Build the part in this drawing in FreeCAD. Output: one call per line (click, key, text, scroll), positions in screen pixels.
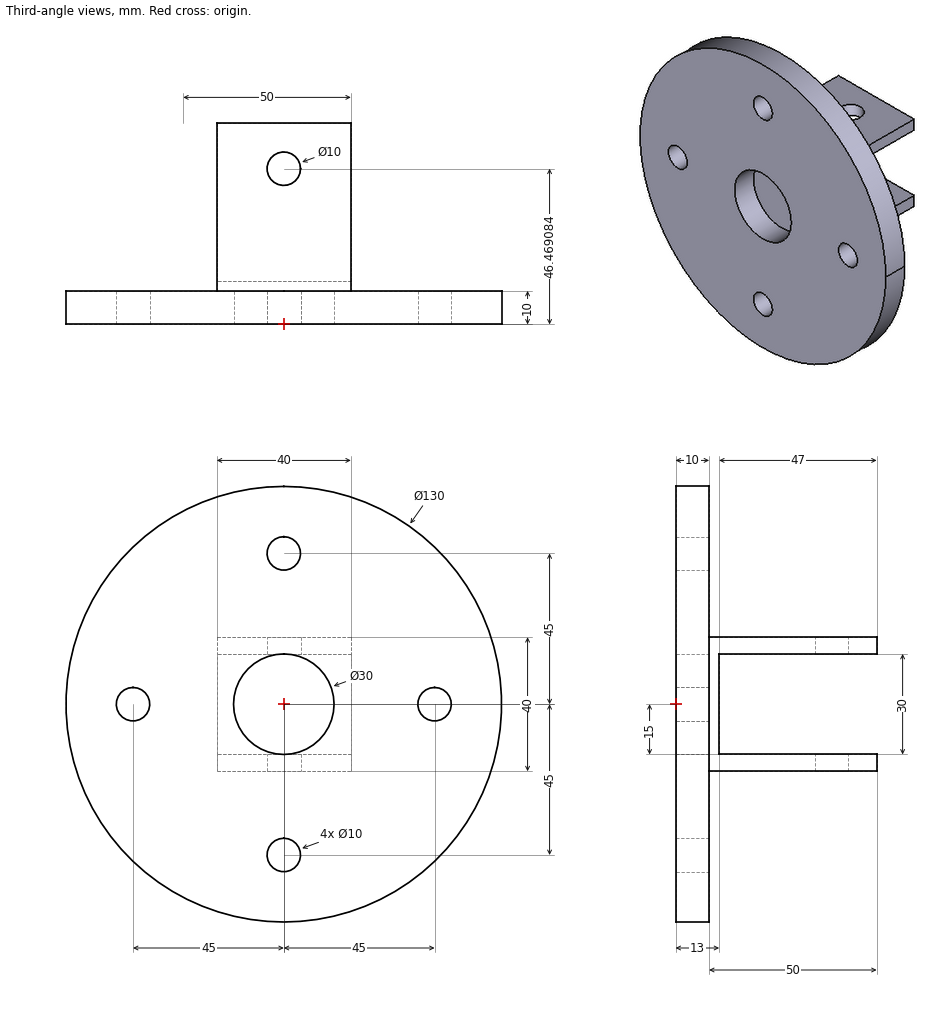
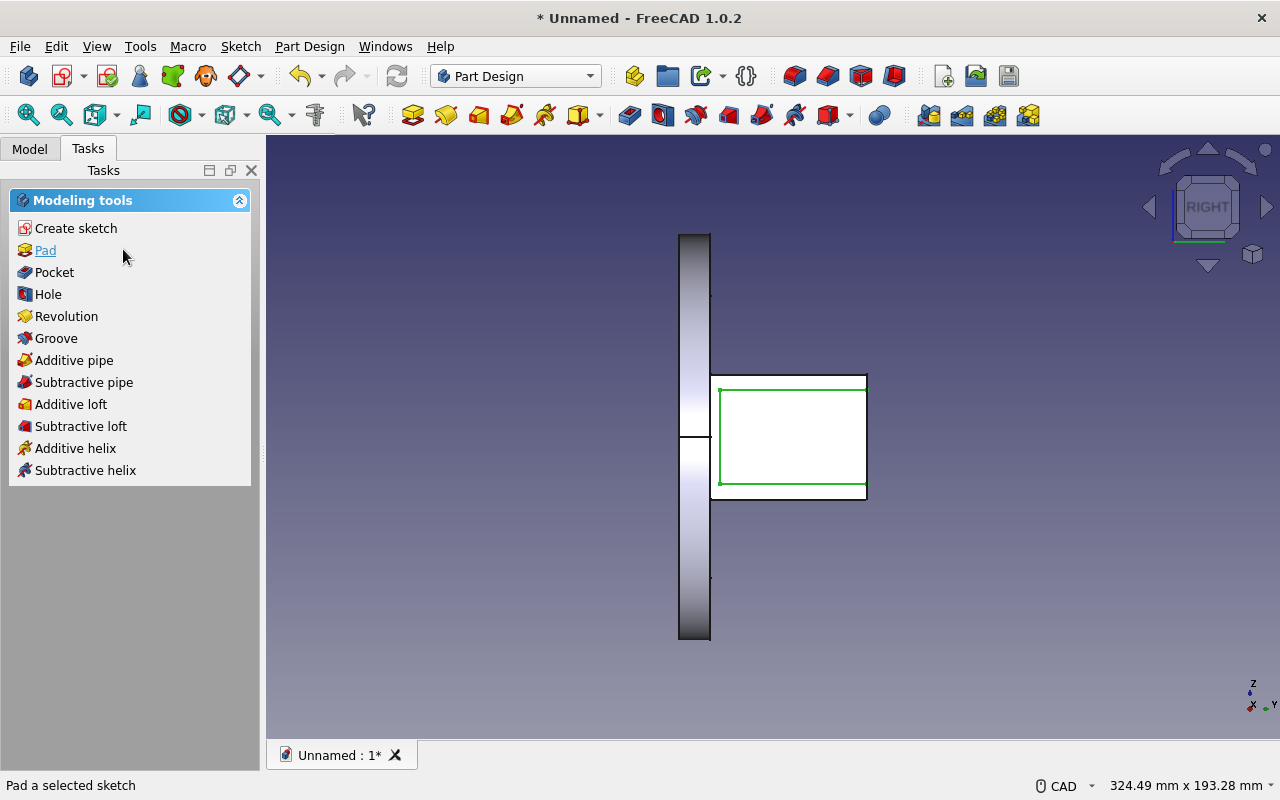
click(630, 116)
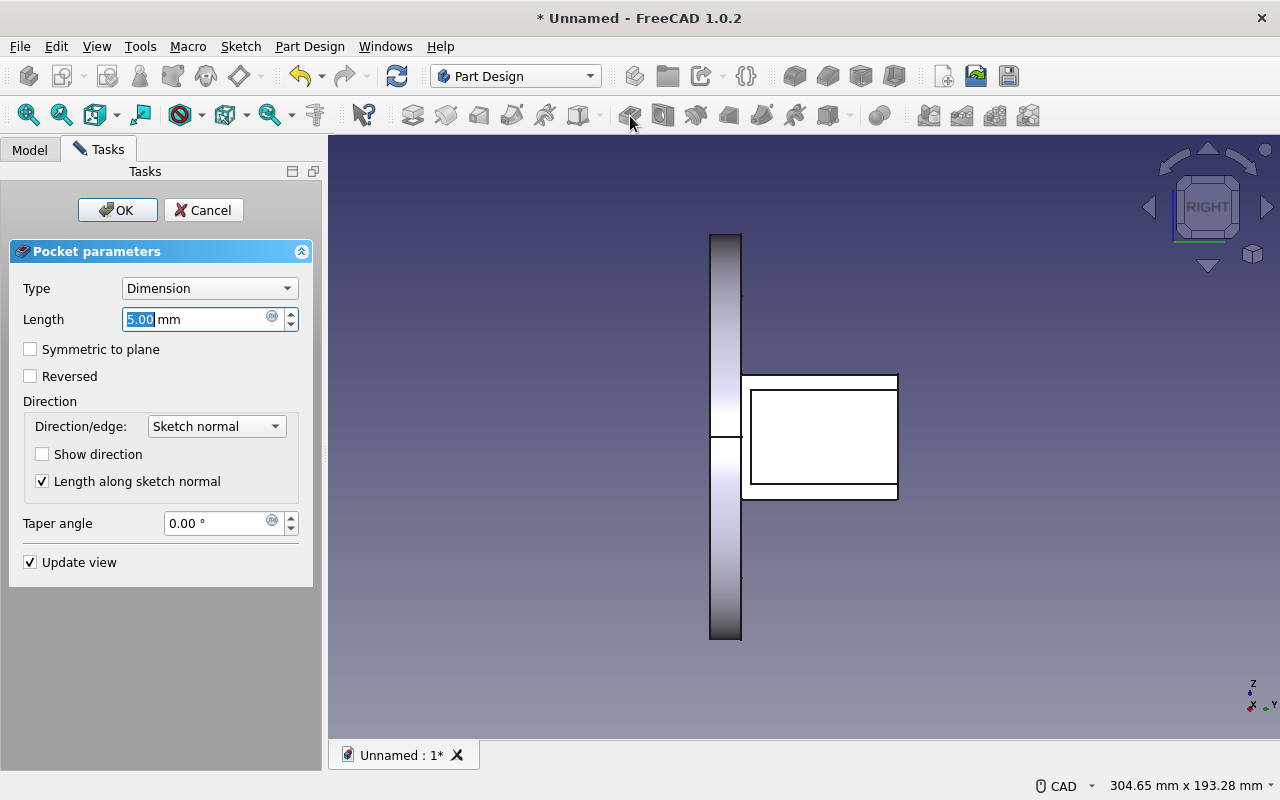
text(50)
key(Tab)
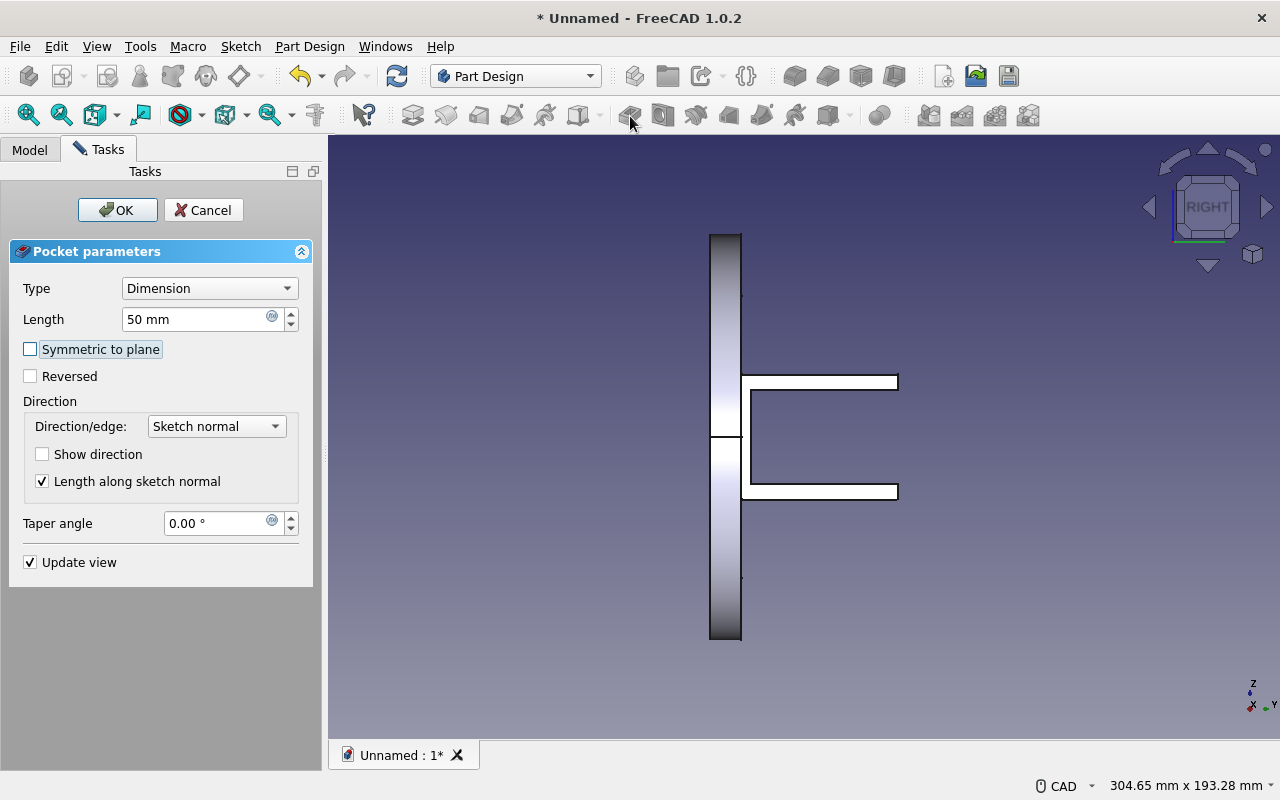
click(118, 210)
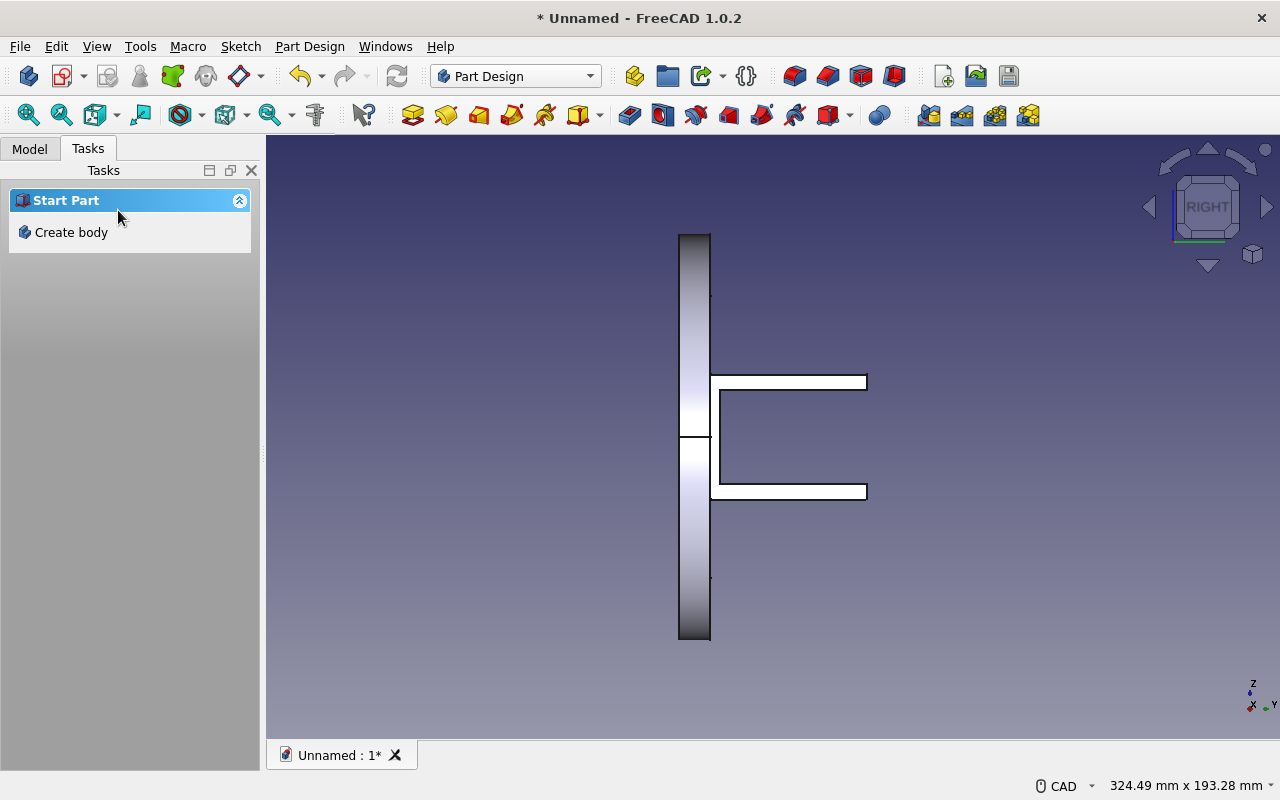
key(0)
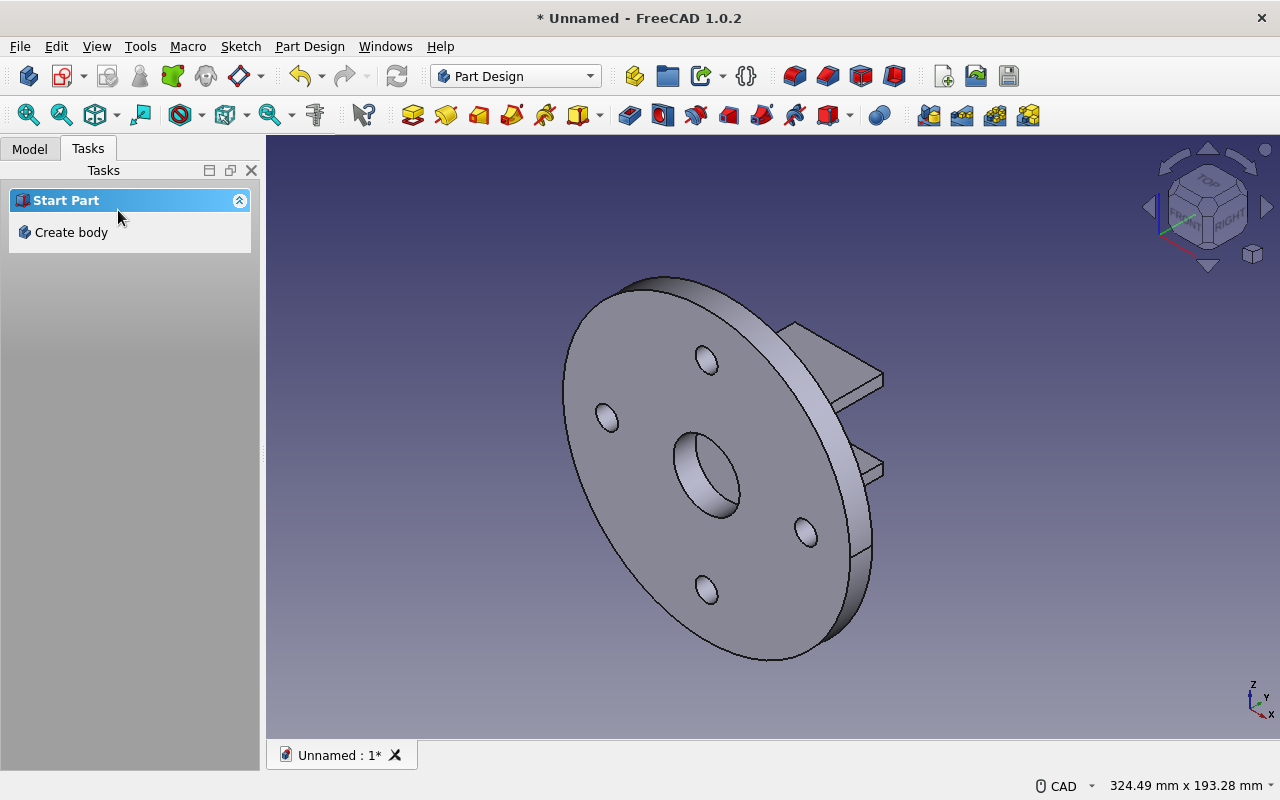
key(2)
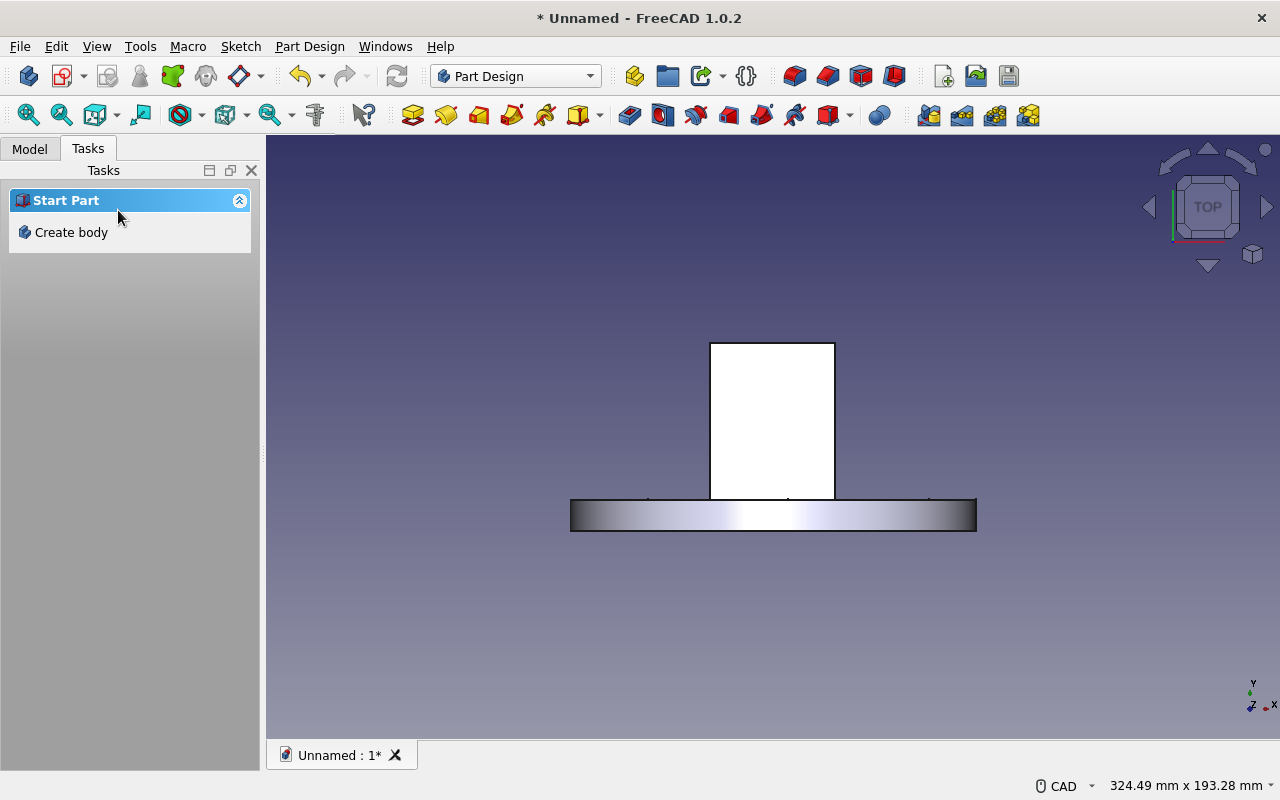
click(29, 116)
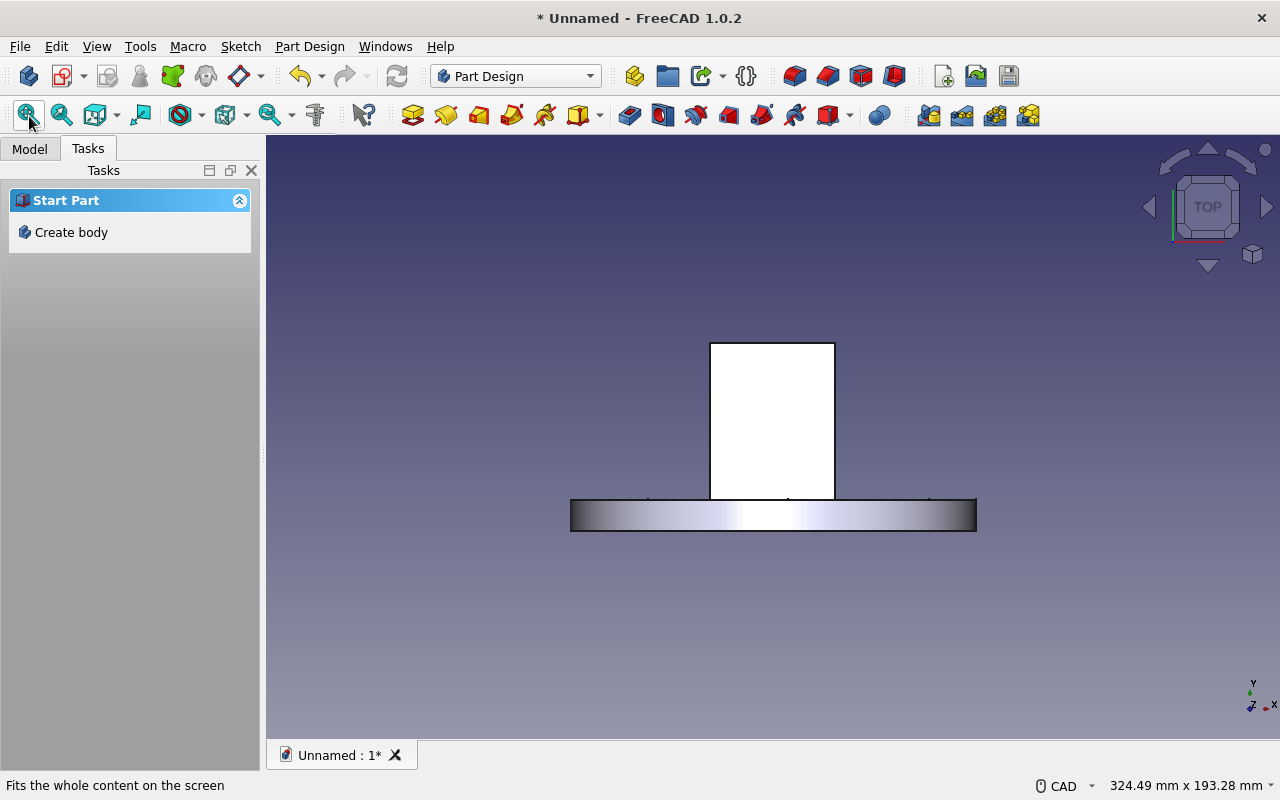
click(773, 420)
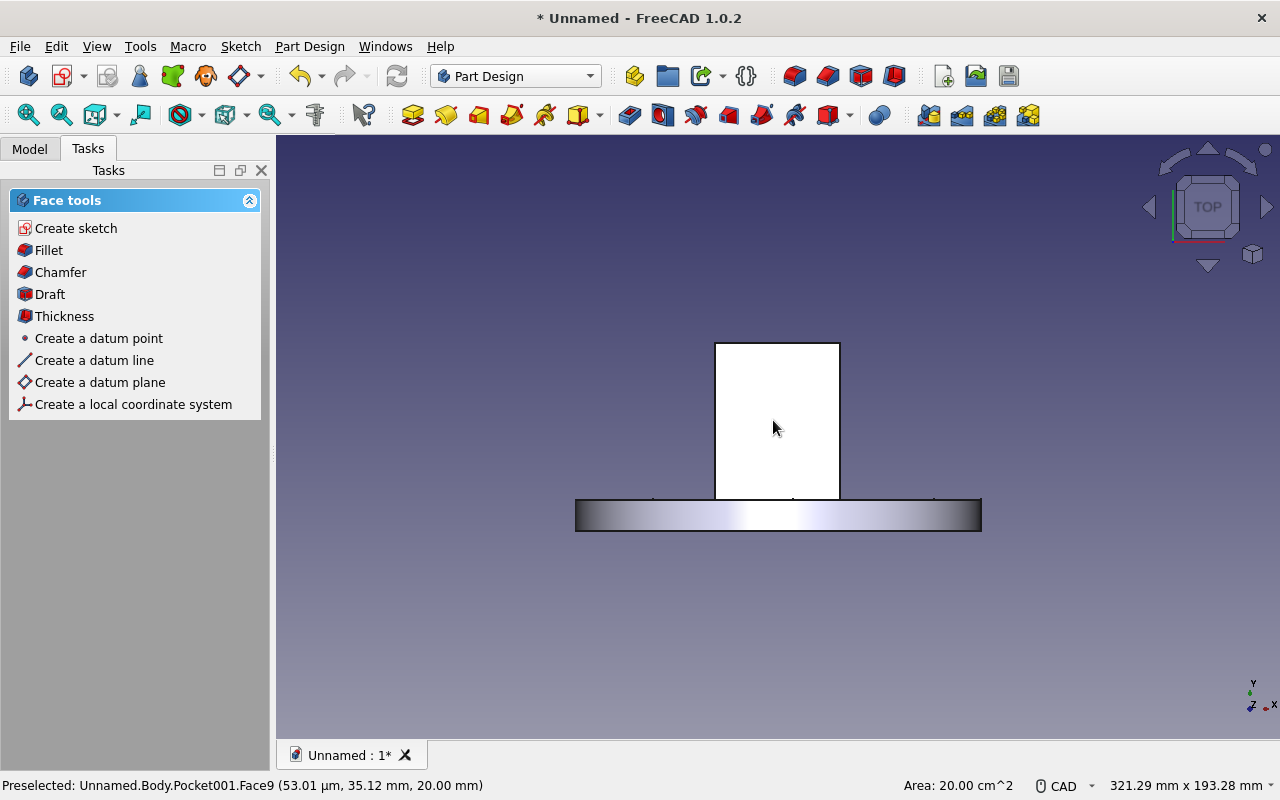
click(62, 76)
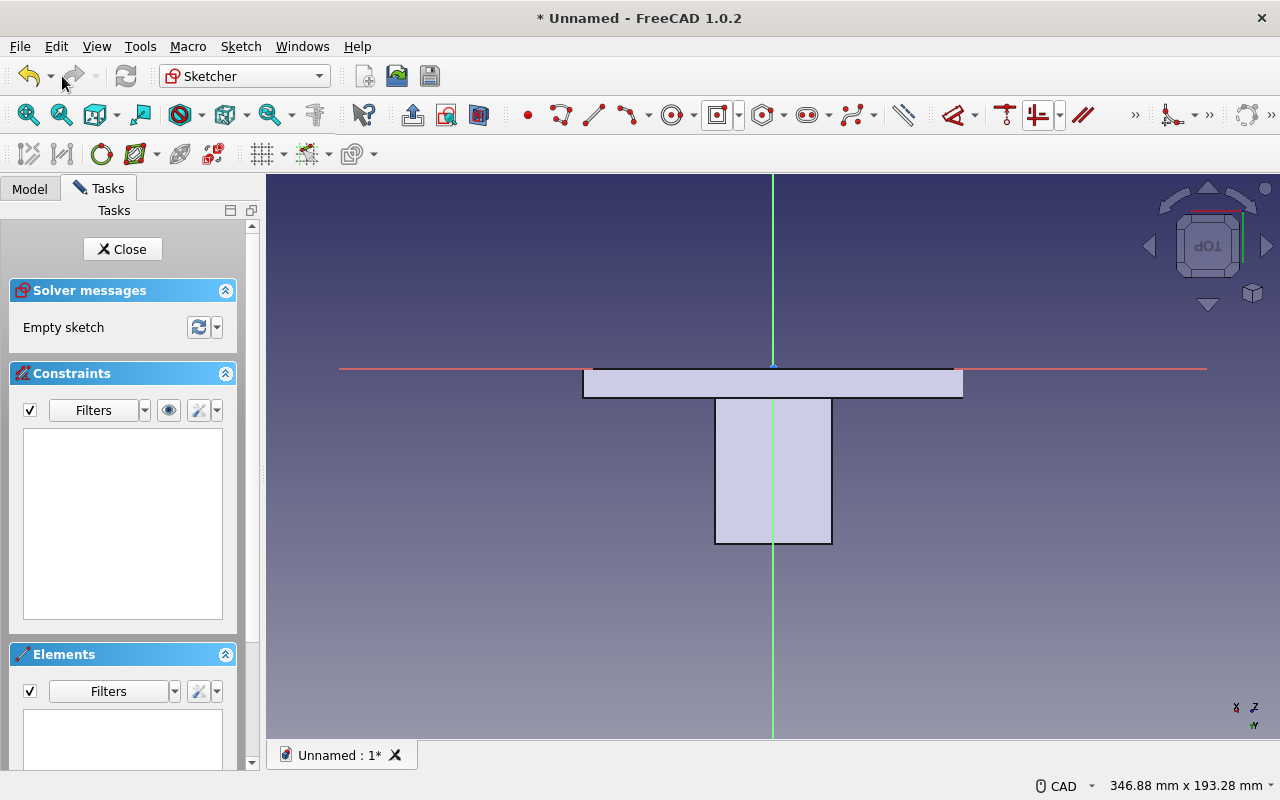
scroll(779, 509, up, 13)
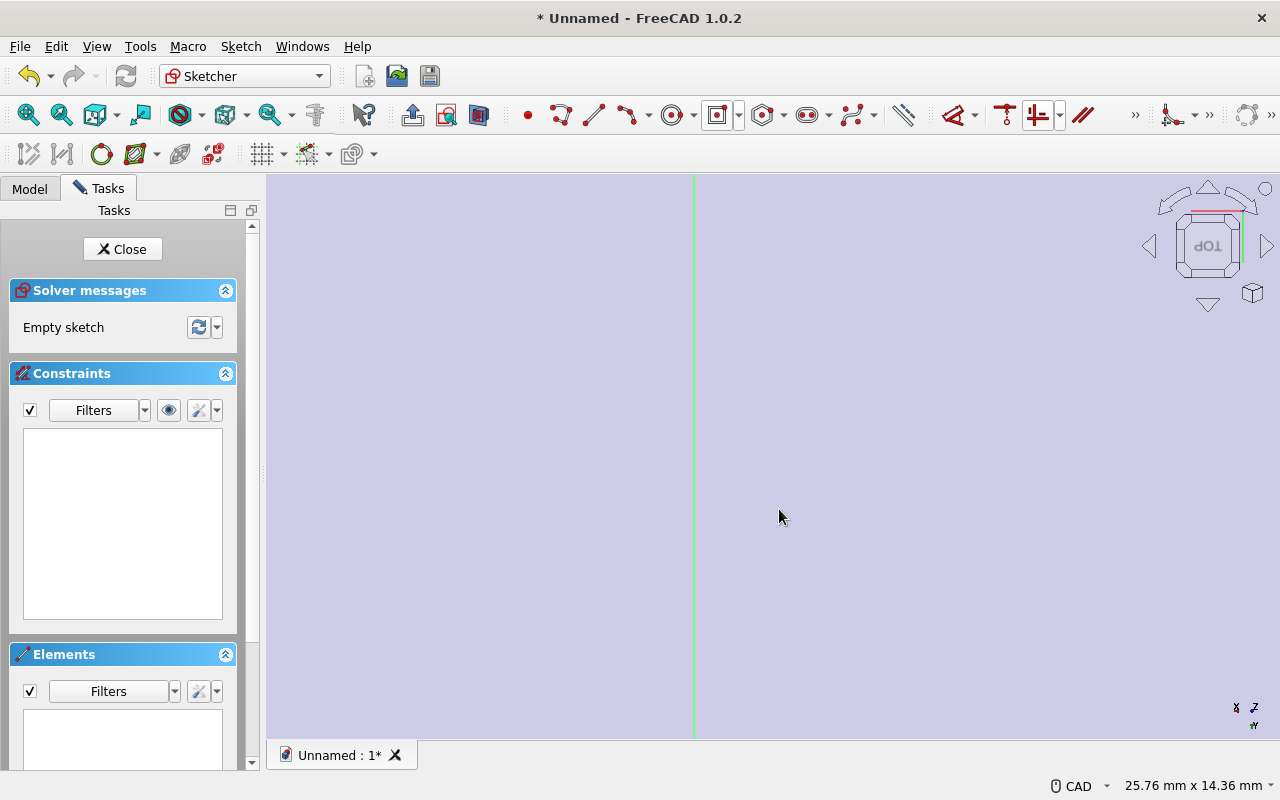
key(g)
key(c)